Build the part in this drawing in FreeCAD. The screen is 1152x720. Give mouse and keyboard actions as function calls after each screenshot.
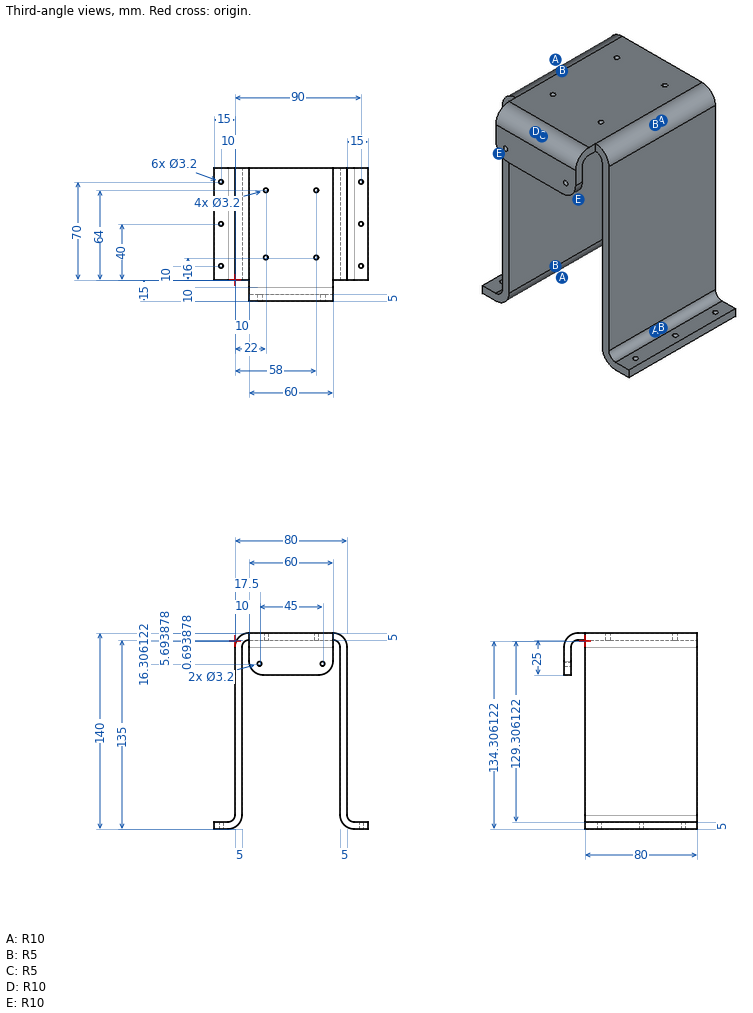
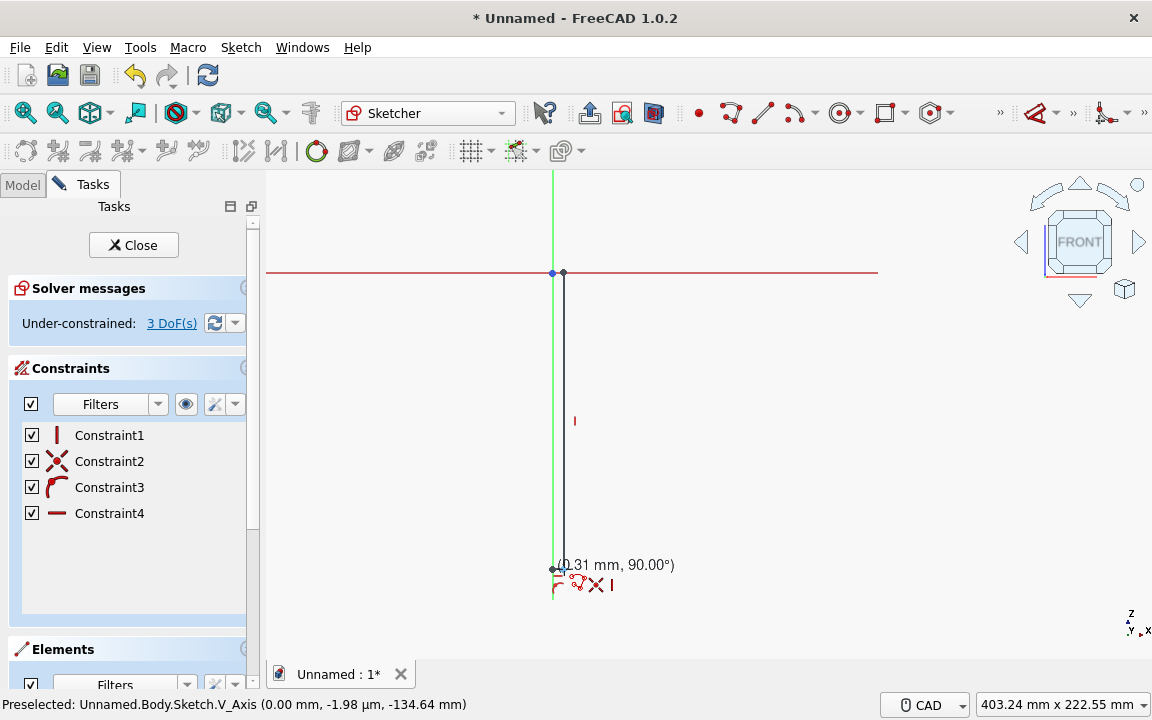
scroll(553, 261, up, 2)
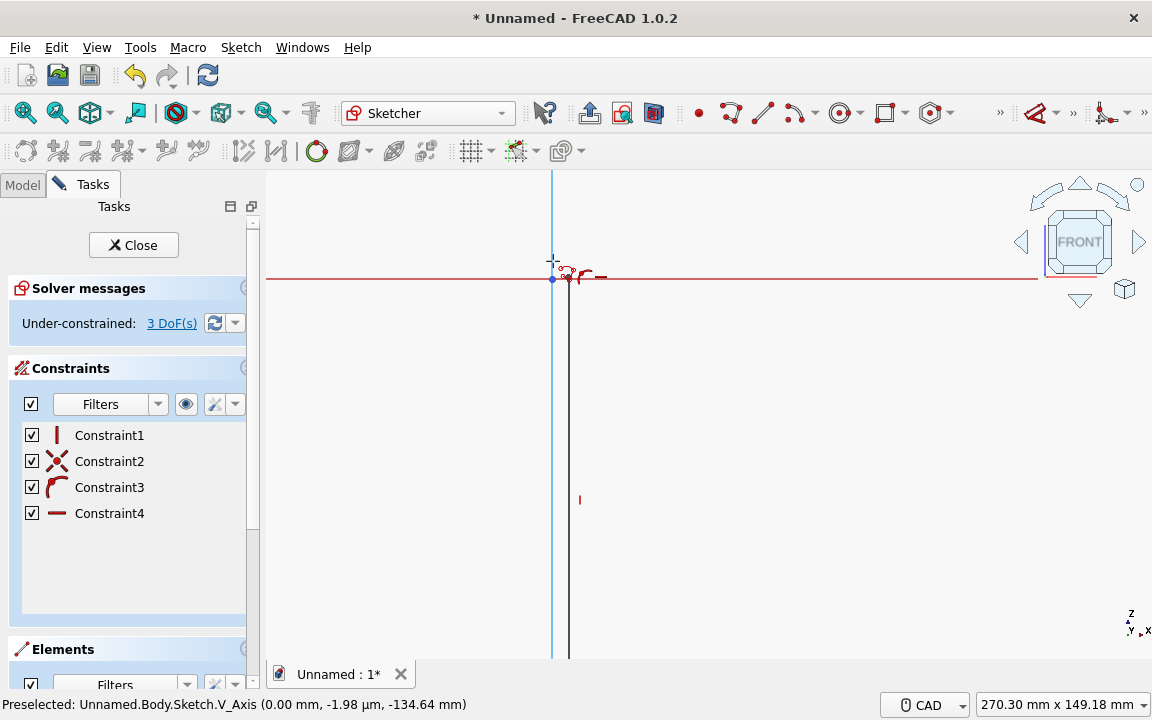
click(561, 261)
click(815, 261)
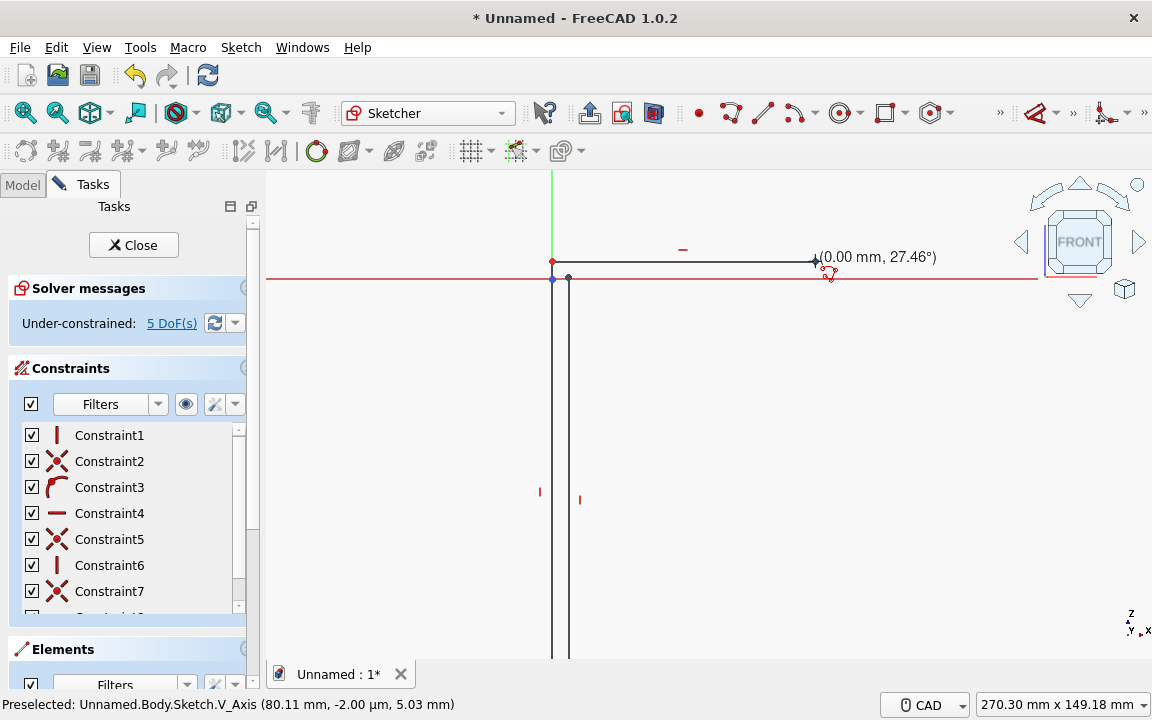
scroll(553, 260, down, 2)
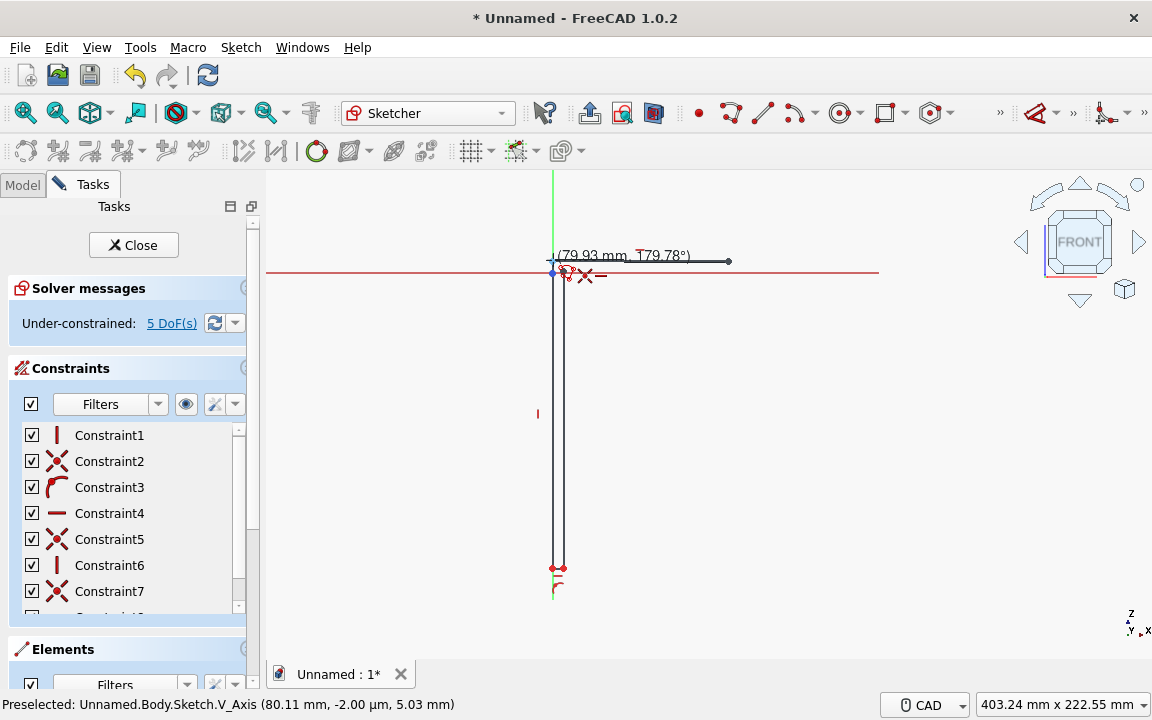
click(729, 568)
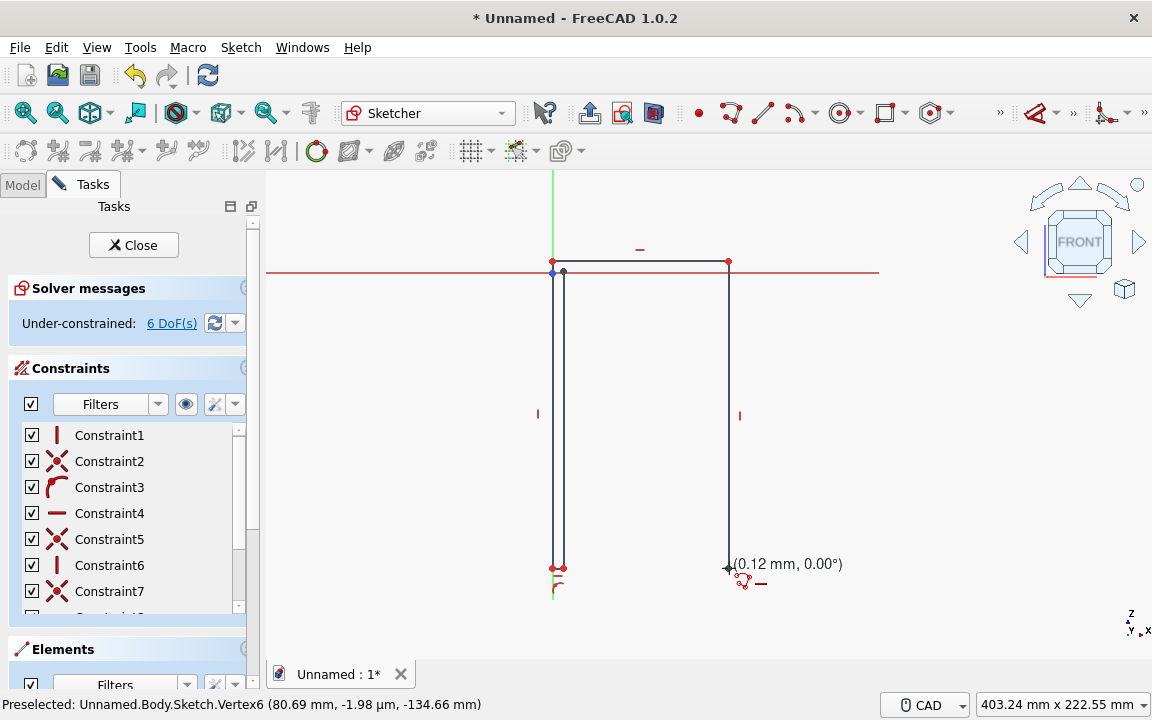
scroll(717, 568, up, 2)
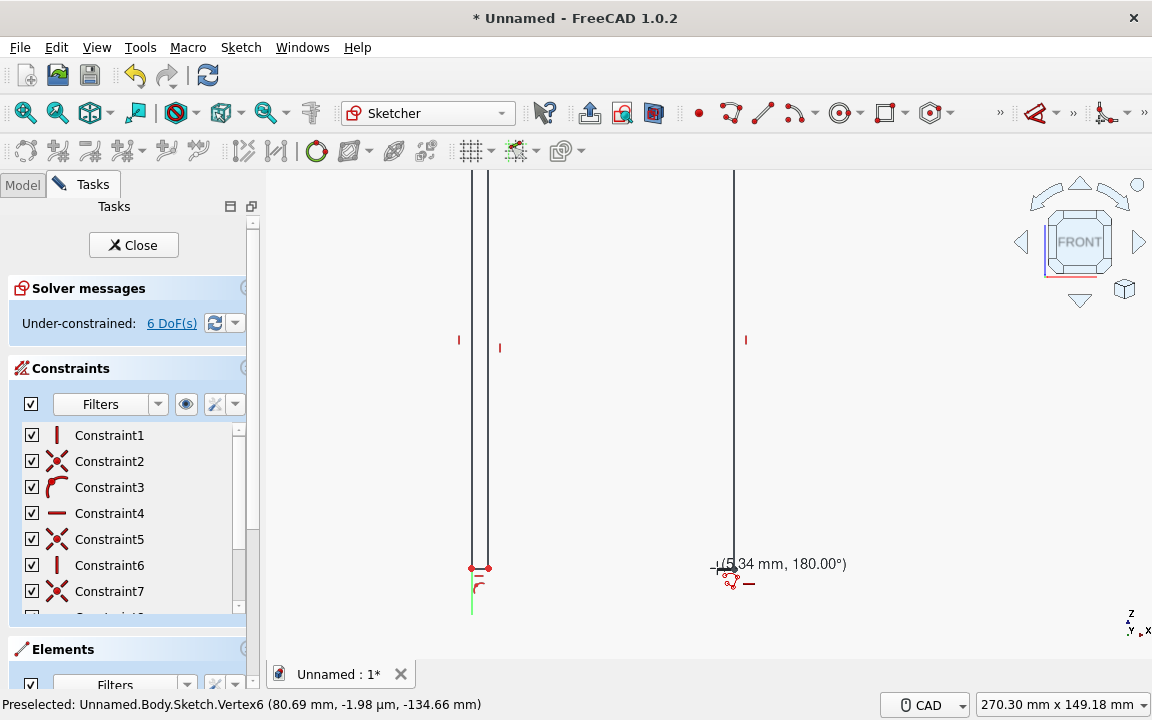
click(717, 568)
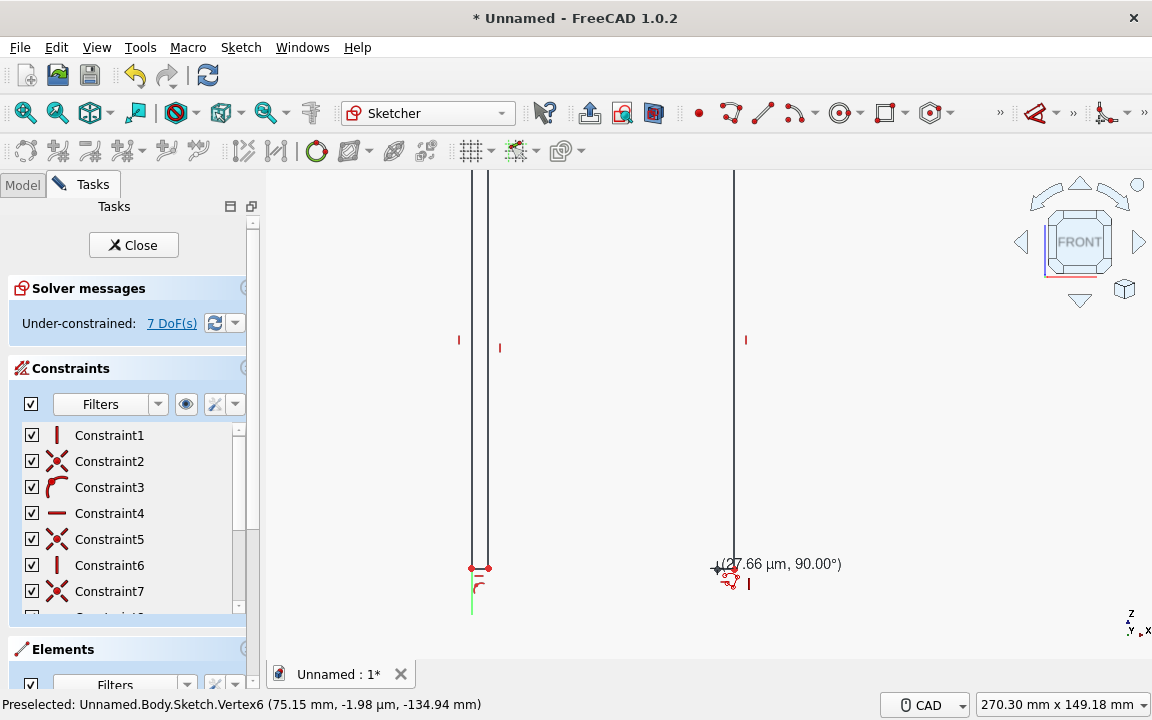
scroll(717, 569, down, 2)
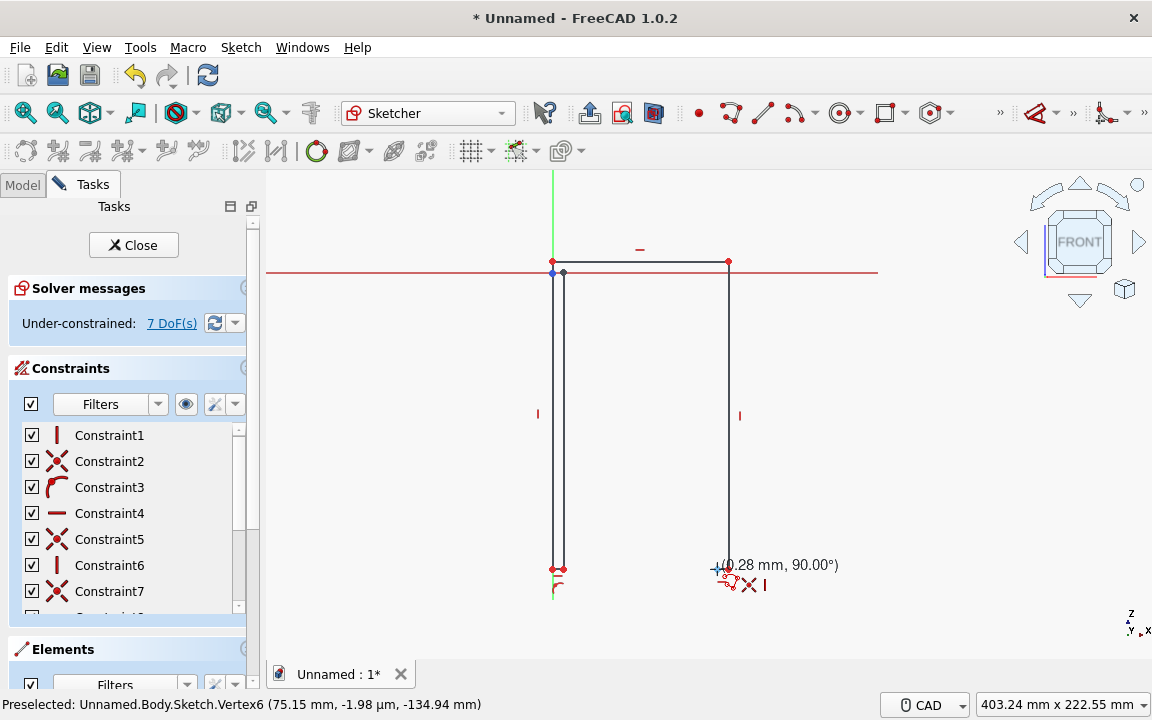
scroll(717, 272, up, 12)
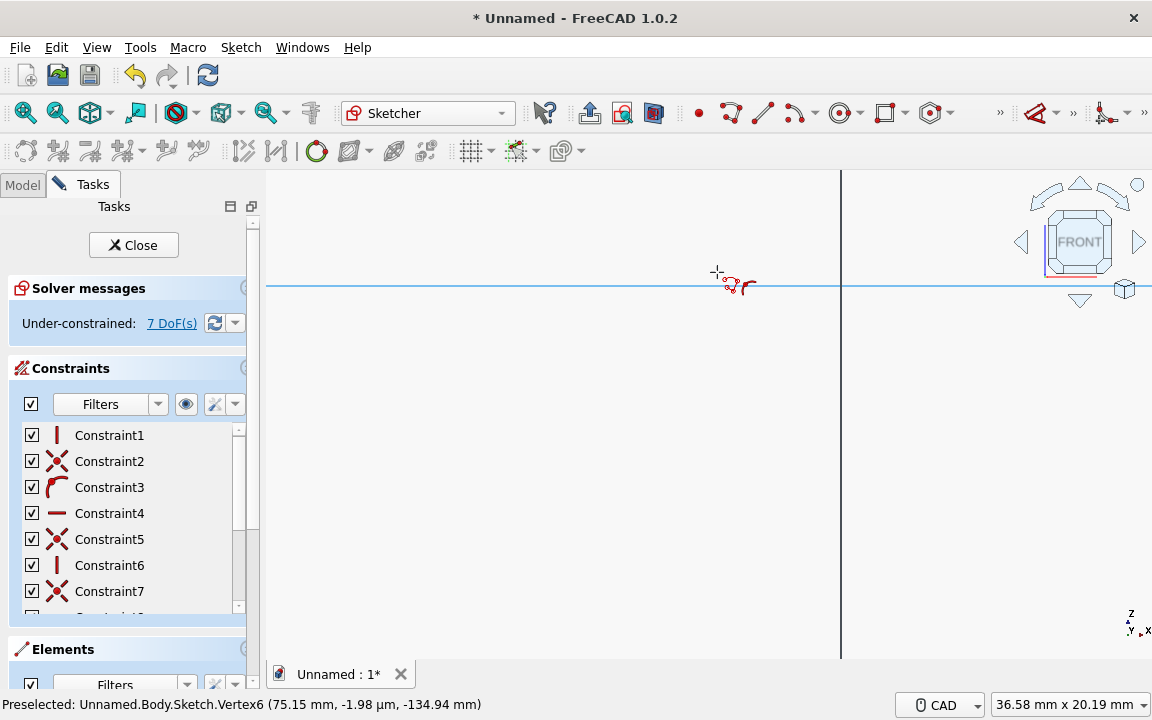
click(714, 269)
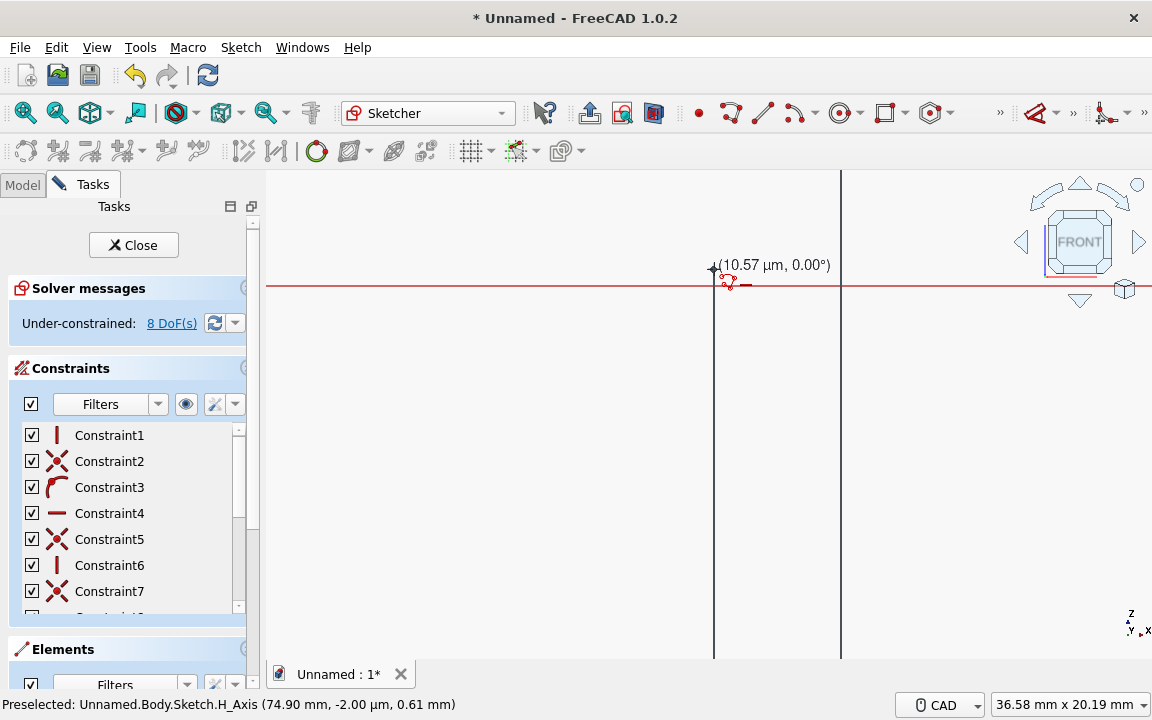
scroll(717, 272, down, 12)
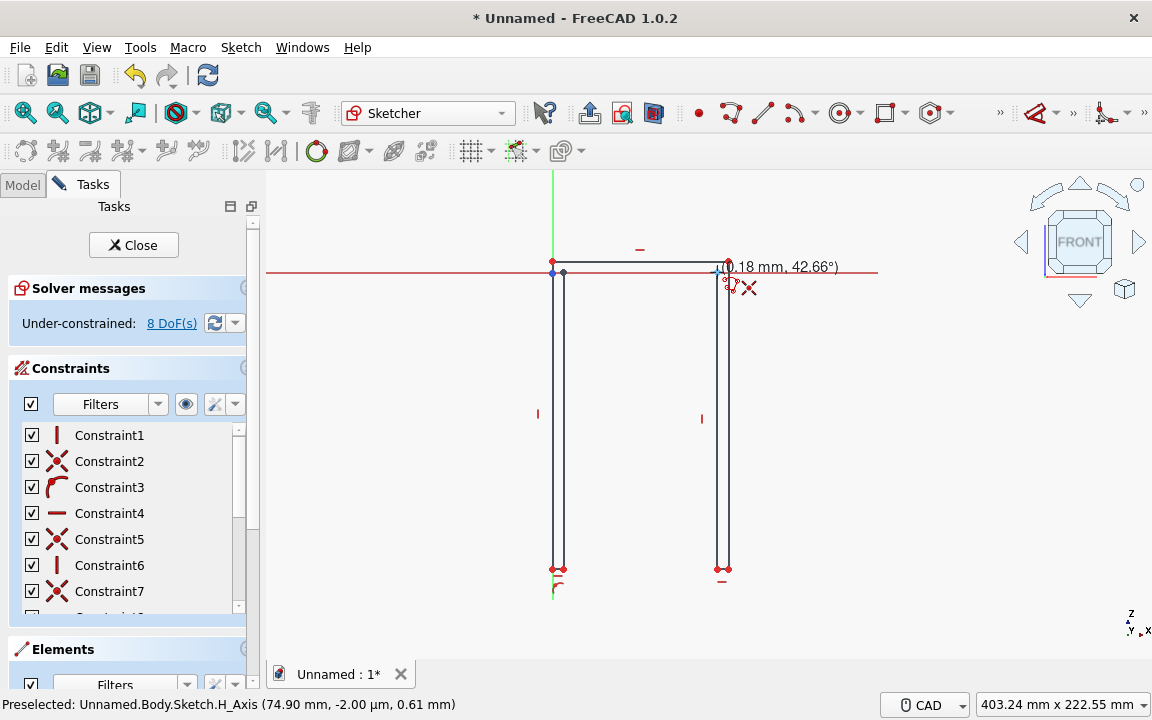
scroll(564, 272, up, 12)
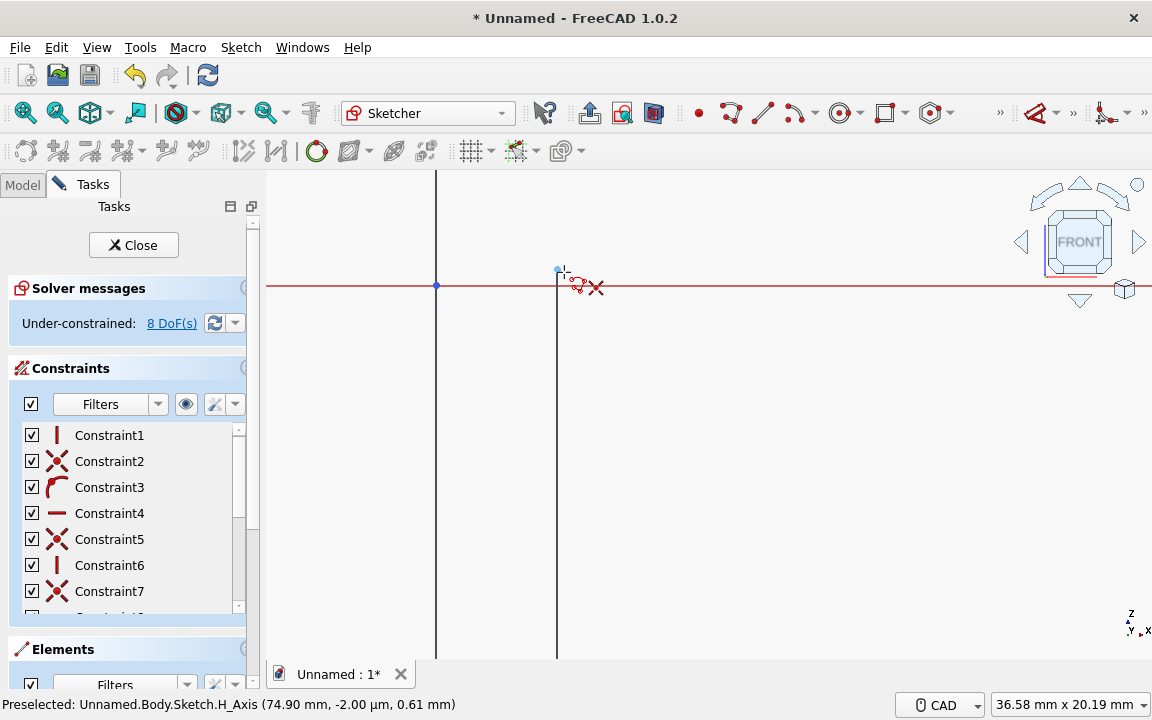
click(557, 270)
key(Escape)
key(Escape)